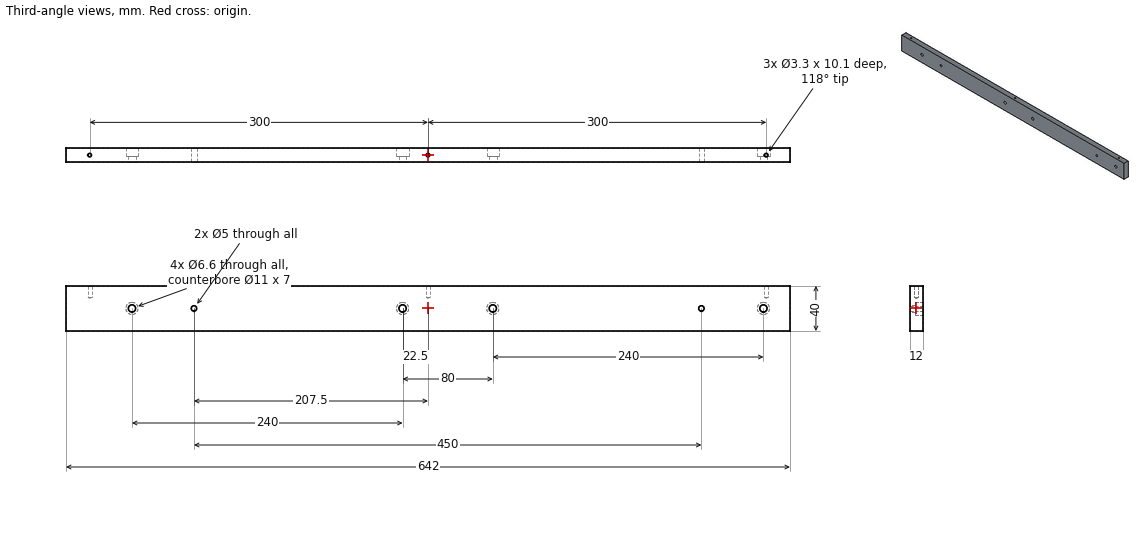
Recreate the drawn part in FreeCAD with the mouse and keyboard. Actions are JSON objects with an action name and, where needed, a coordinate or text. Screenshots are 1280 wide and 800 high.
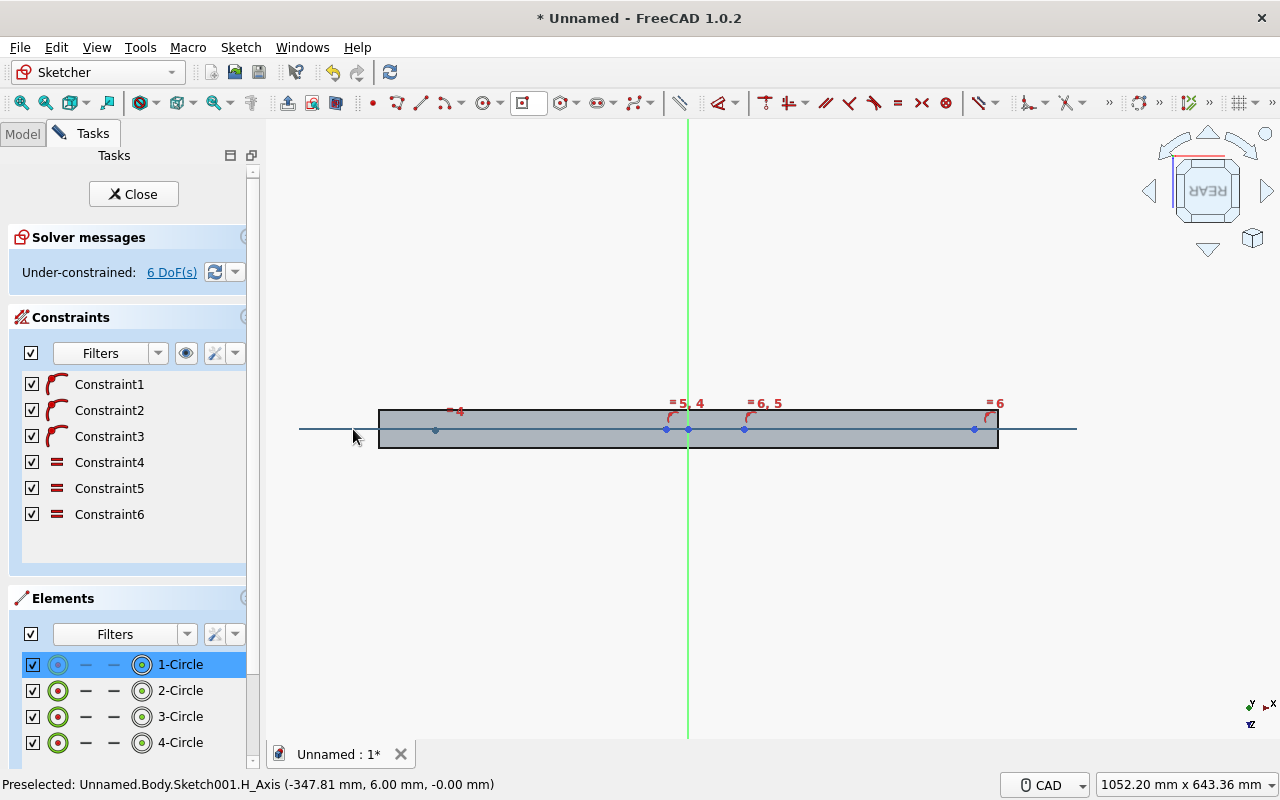
{"action": "left_click", "coordinate": [766, 104]}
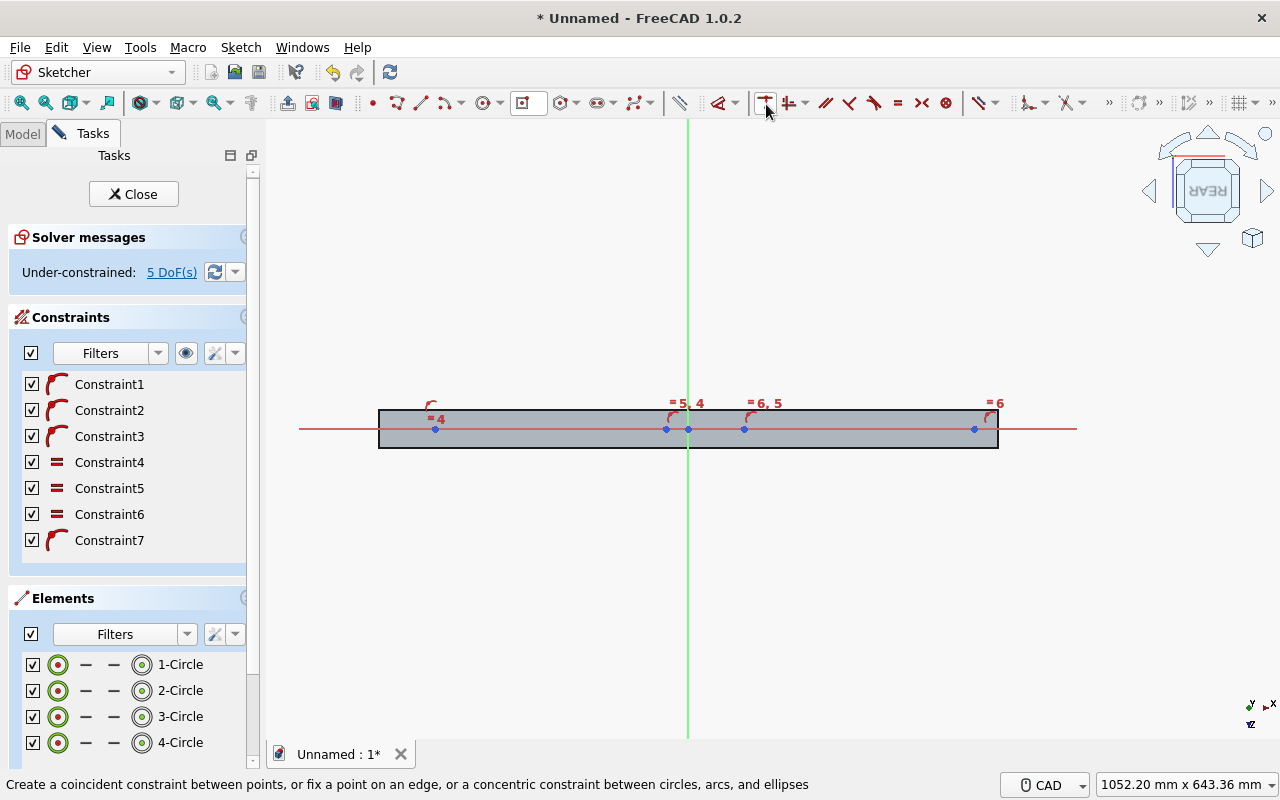
{"action": "left_click", "coordinate": [718, 104]}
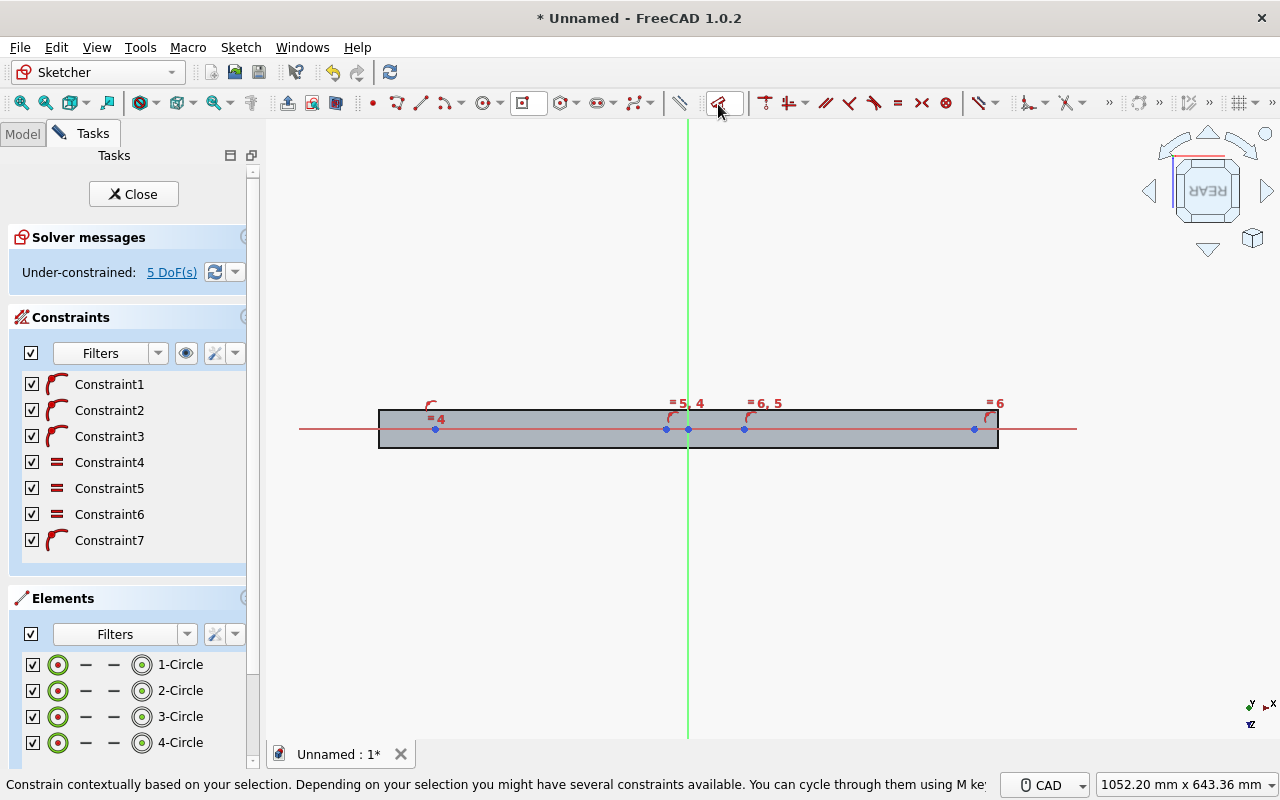
{"action": "scroll", "coordinate": [435, 427], "scroll_direction": "up", "scroll_amount": 10}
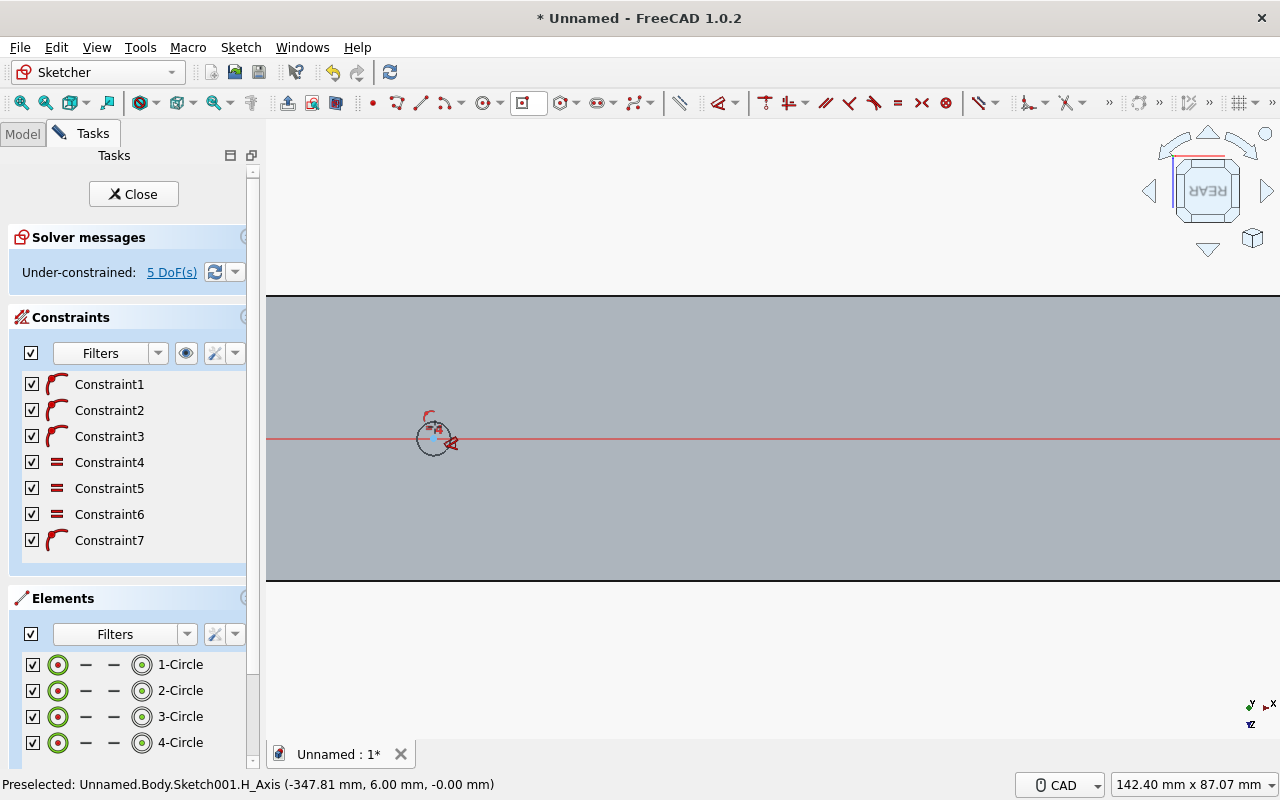
{"action": "left_click", "coordinate": [434, 422]}
{"action": "left_click", "coordinate": [434, 390]}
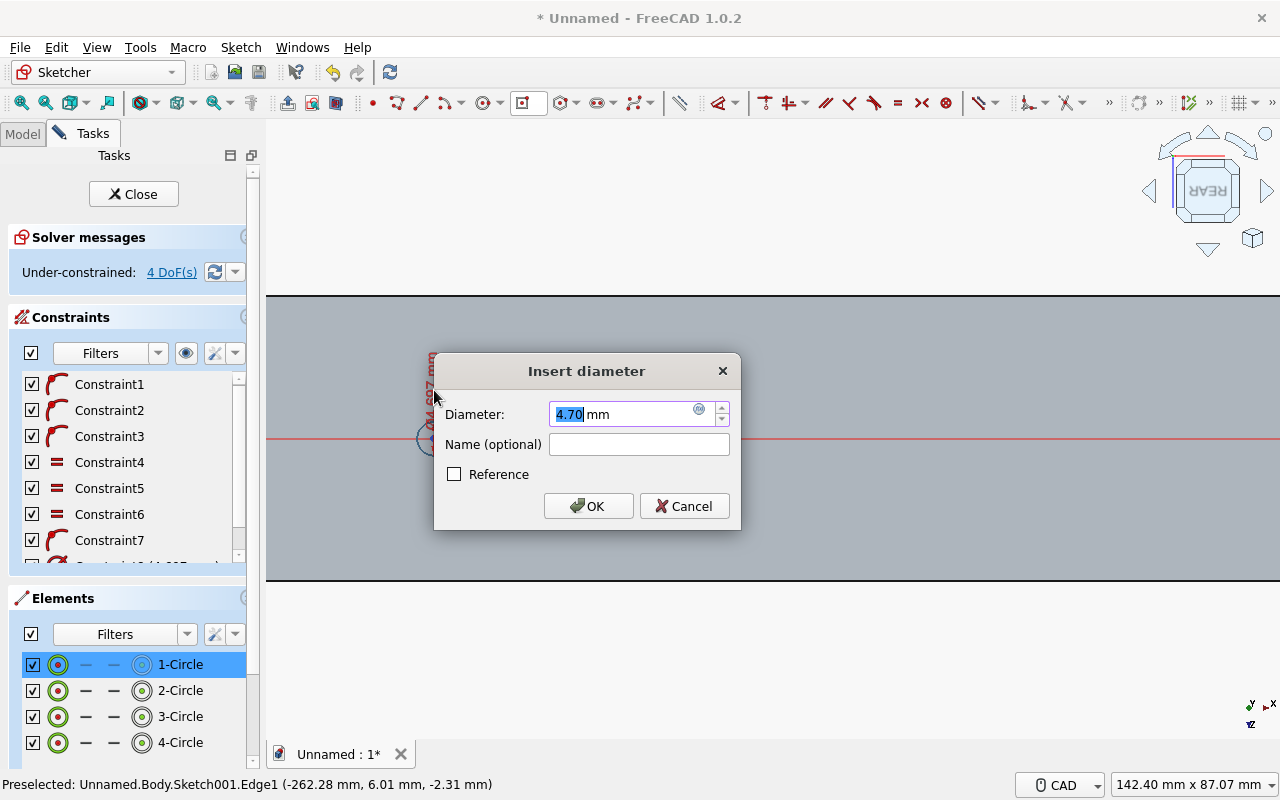
{"action": "type", "text": "6.6"}
{"action": "key", "text": "Return"}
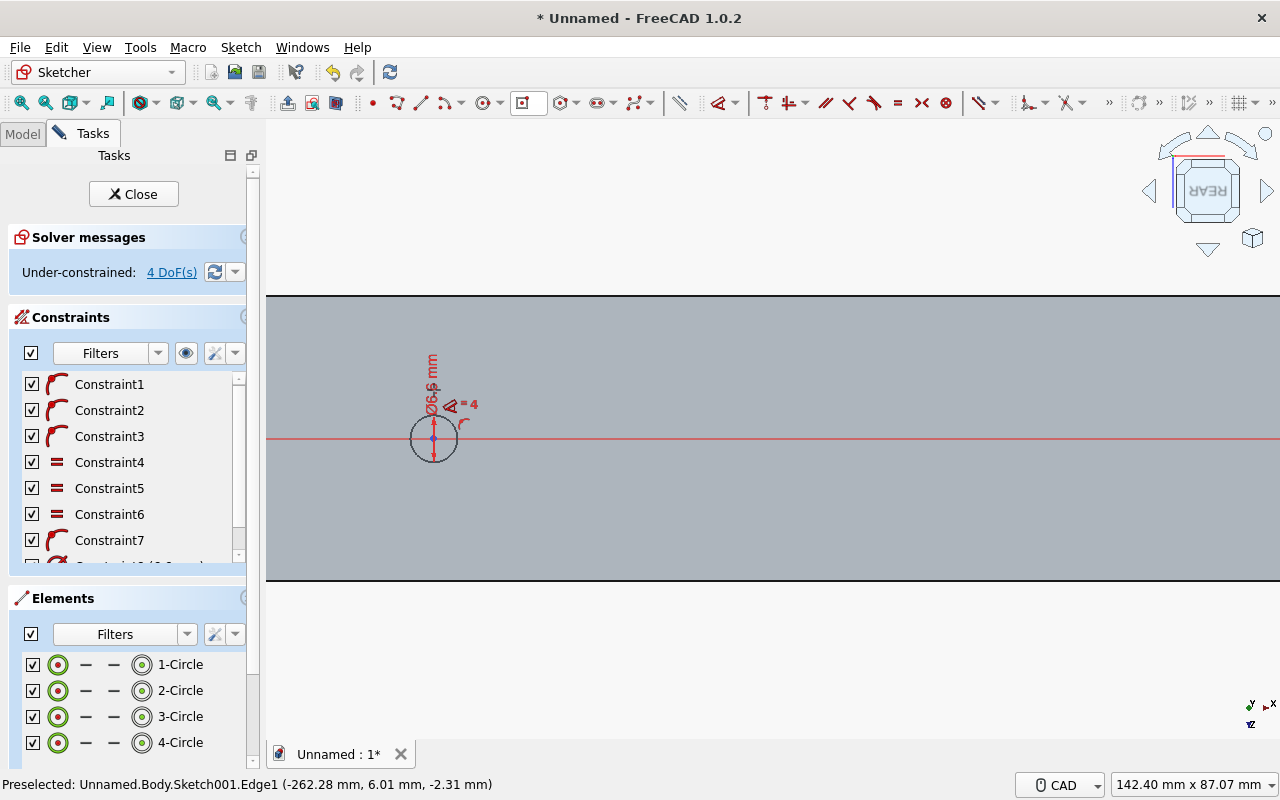
{"action": "scroll", "coordinate": [435, 427], "scroll_direction": "down", "scroll_amount": 10}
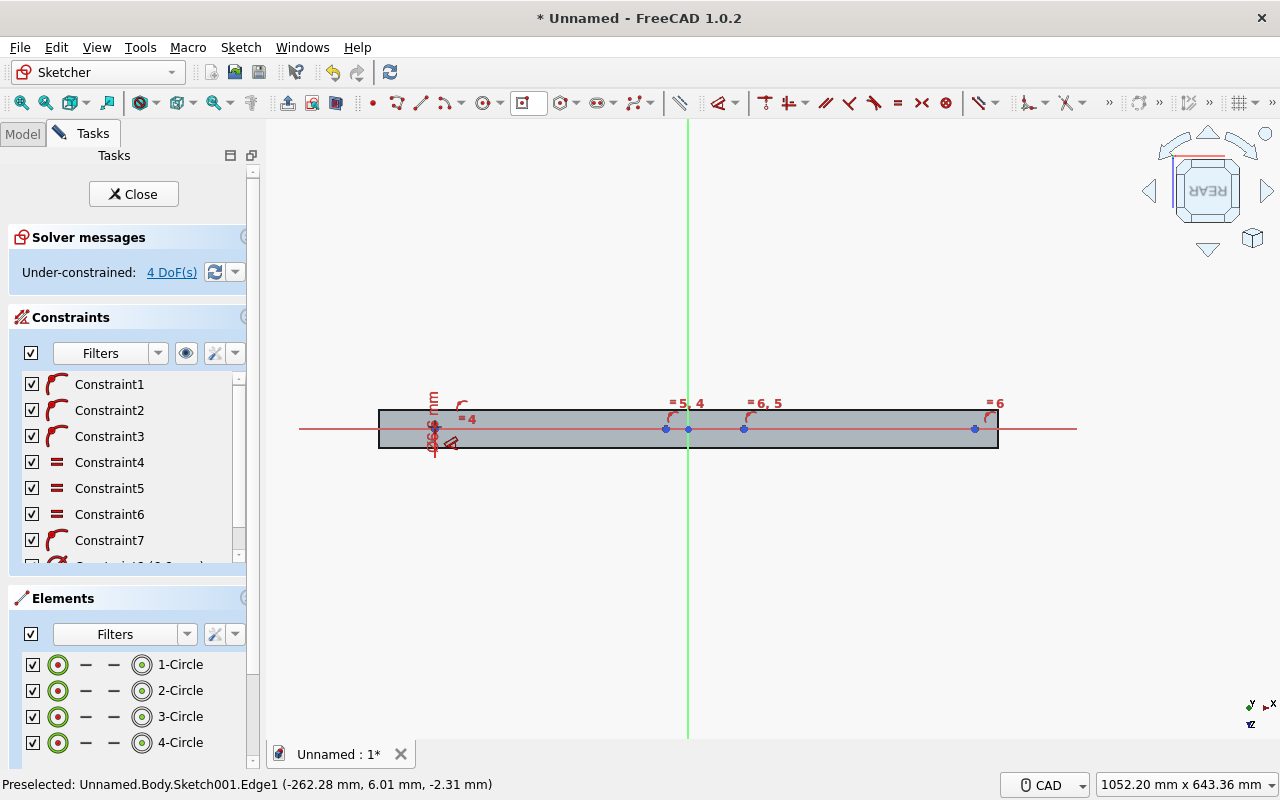
{"action": "left_click", "coordinate": [666, 429]}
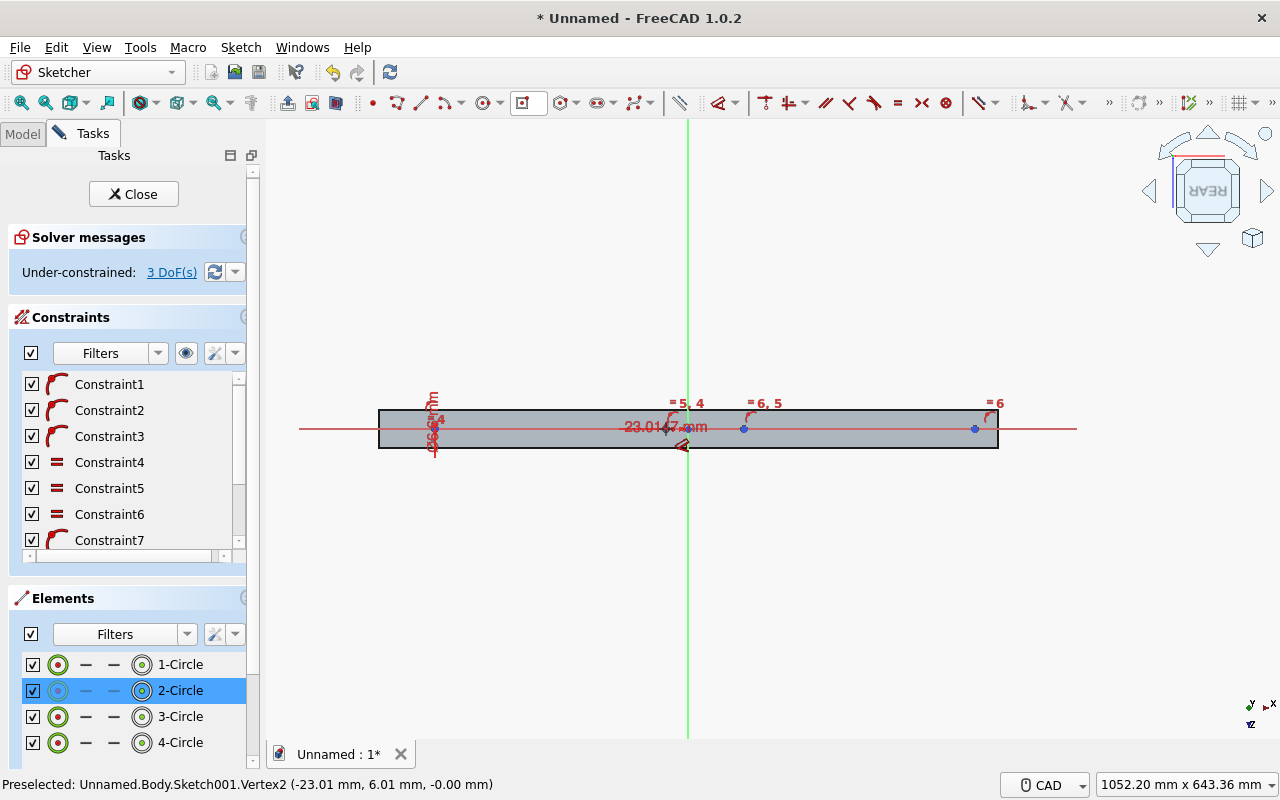
{"action": "left_click", "coordinate": [744, 429]}
{"action": "left_click", "coordinate": [705, 463]}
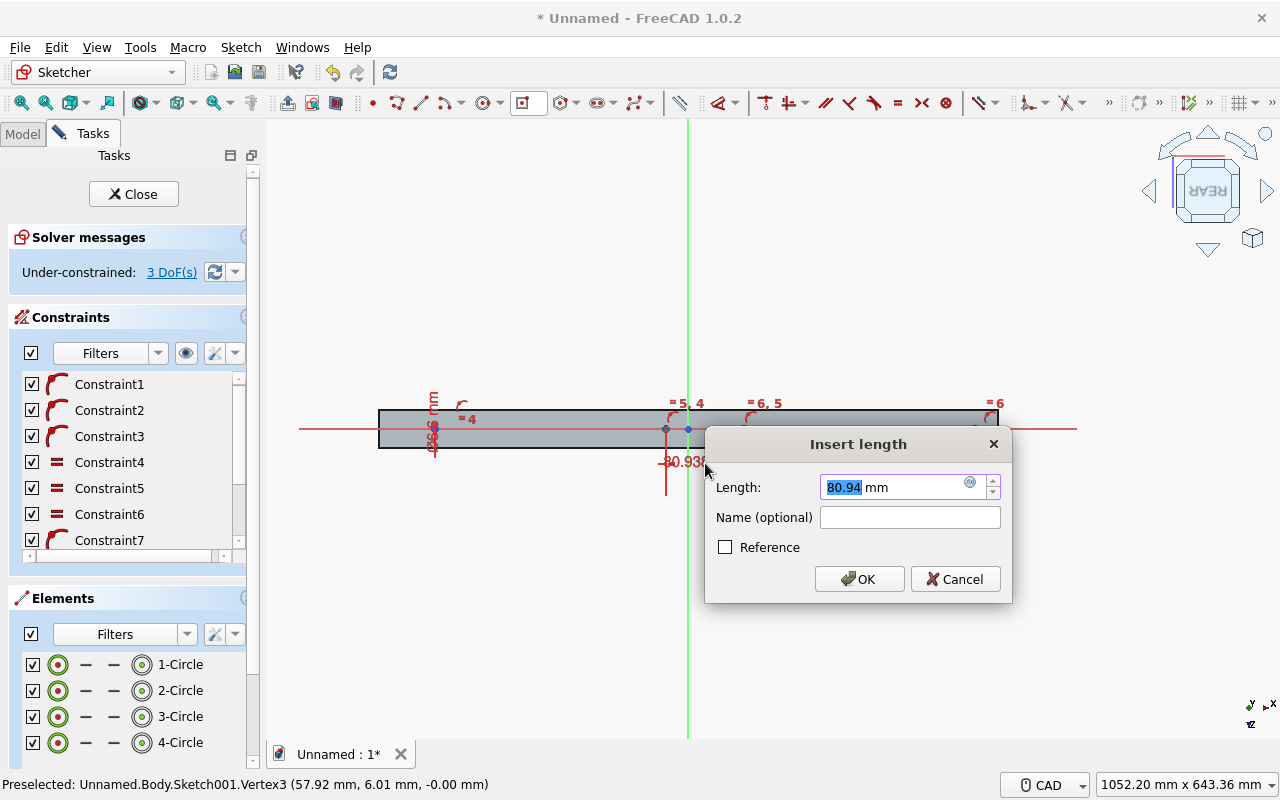
{"action": "type", "text": "80"}
{"action": "key", "text": "Return"}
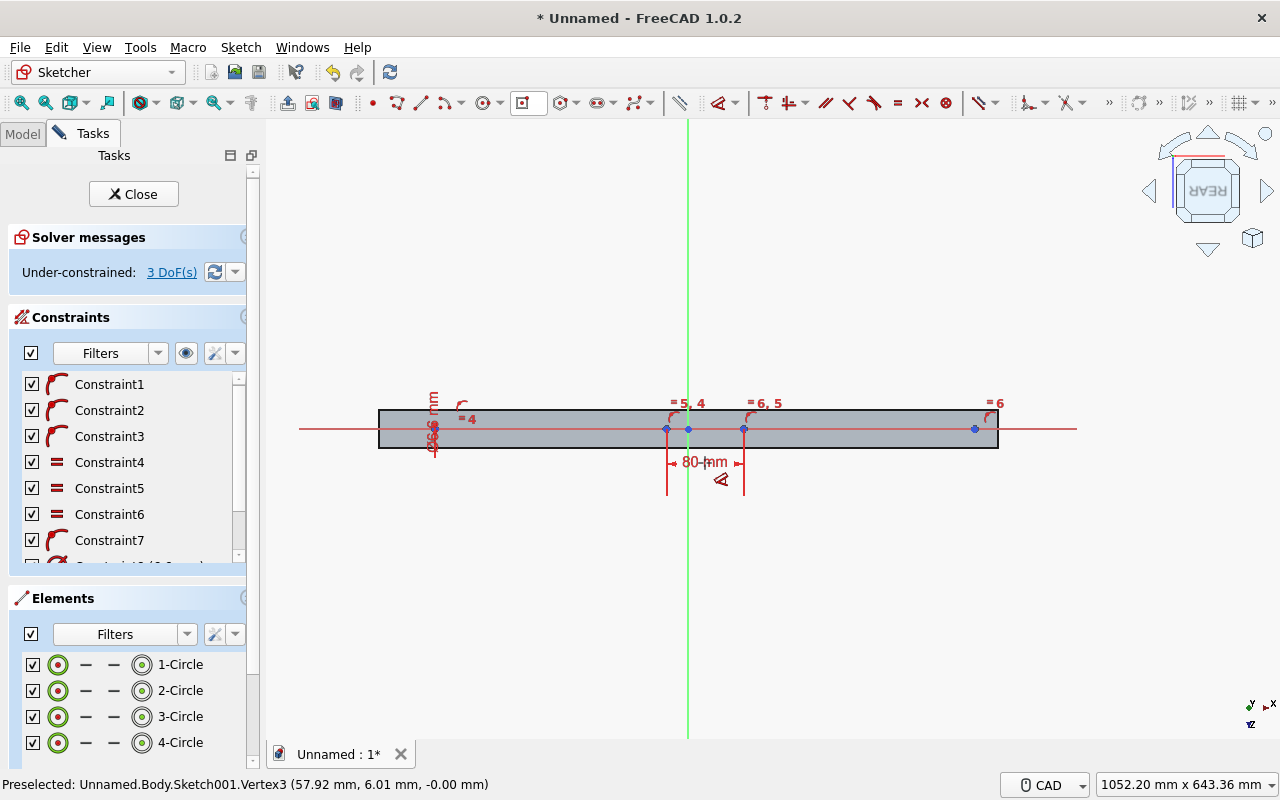
{"action": "scroll", "coordinate": [667, 429], "scroll_direction": "up", "scroll_amount": 4}